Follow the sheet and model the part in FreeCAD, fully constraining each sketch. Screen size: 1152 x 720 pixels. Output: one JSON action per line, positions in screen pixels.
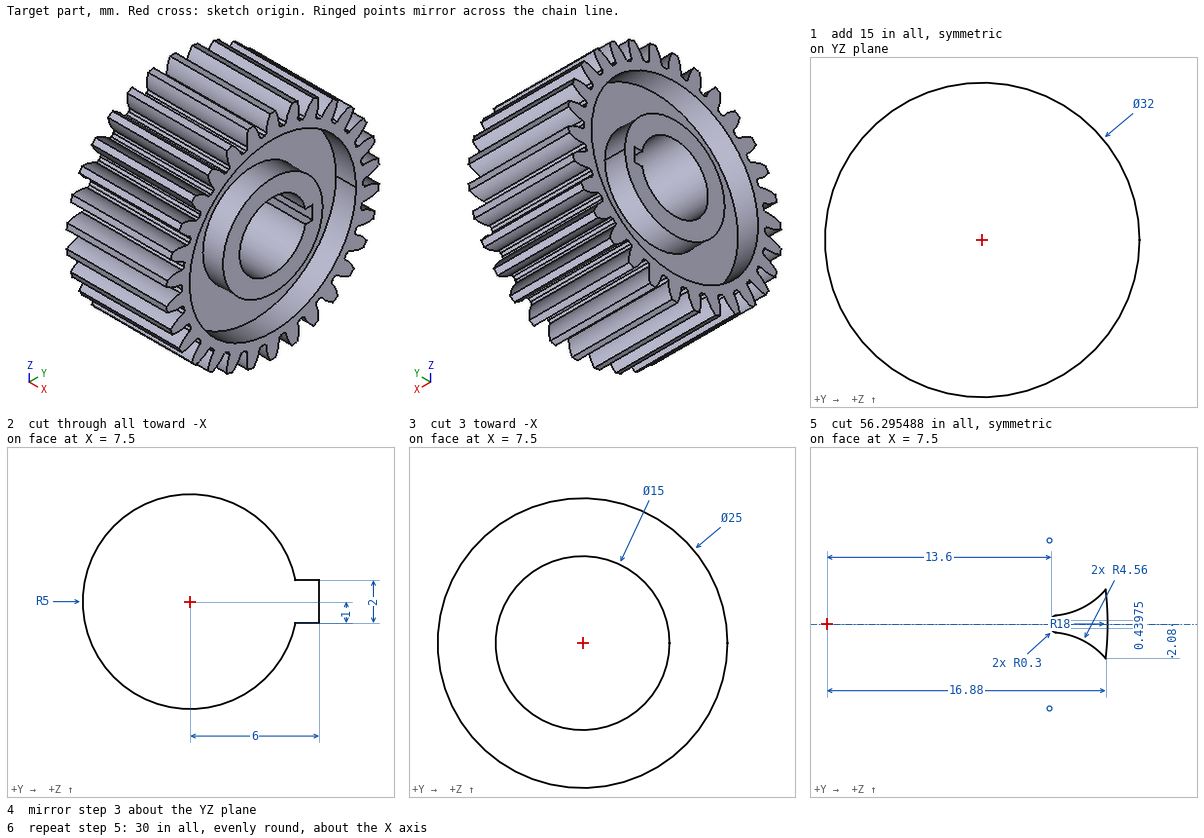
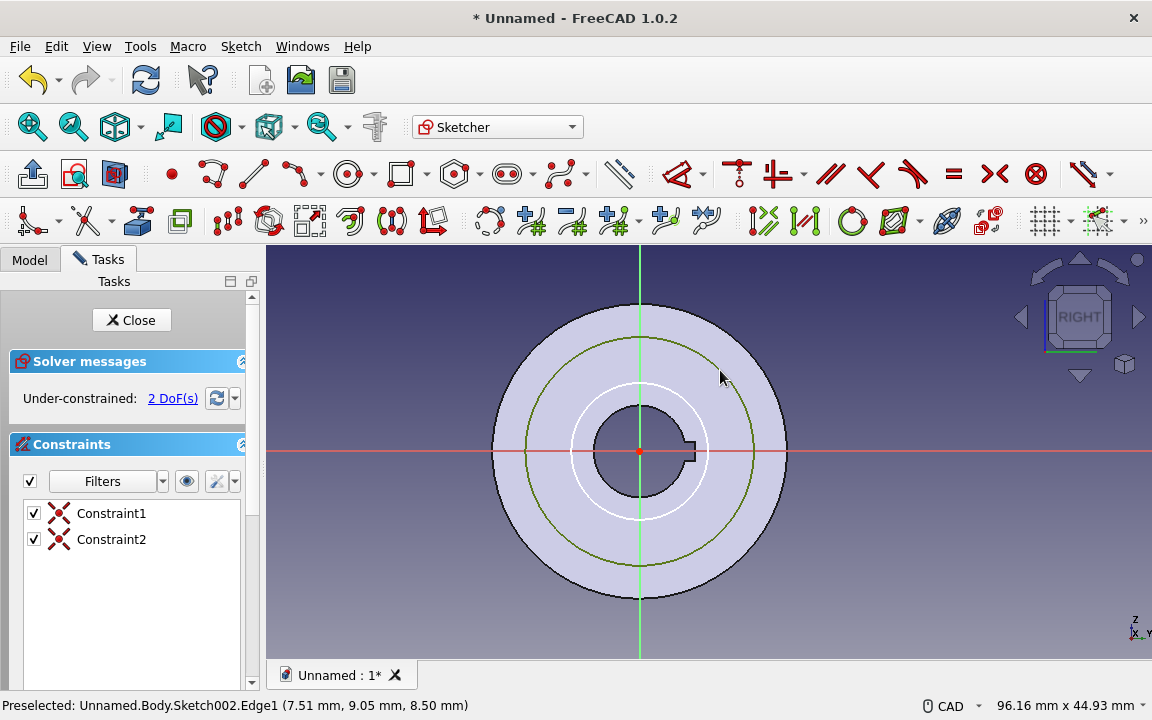
{"action": "left_click", "coordinate": [702, 174]}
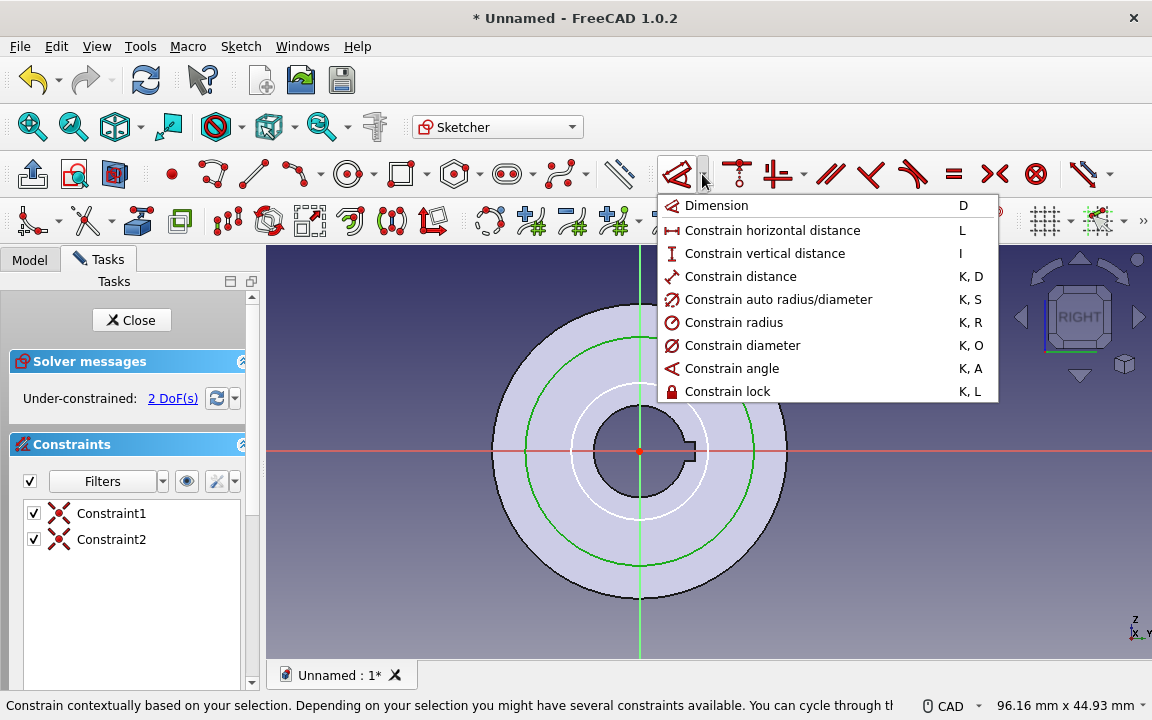
{"action": "left_click", "coordinate": [828, 346]}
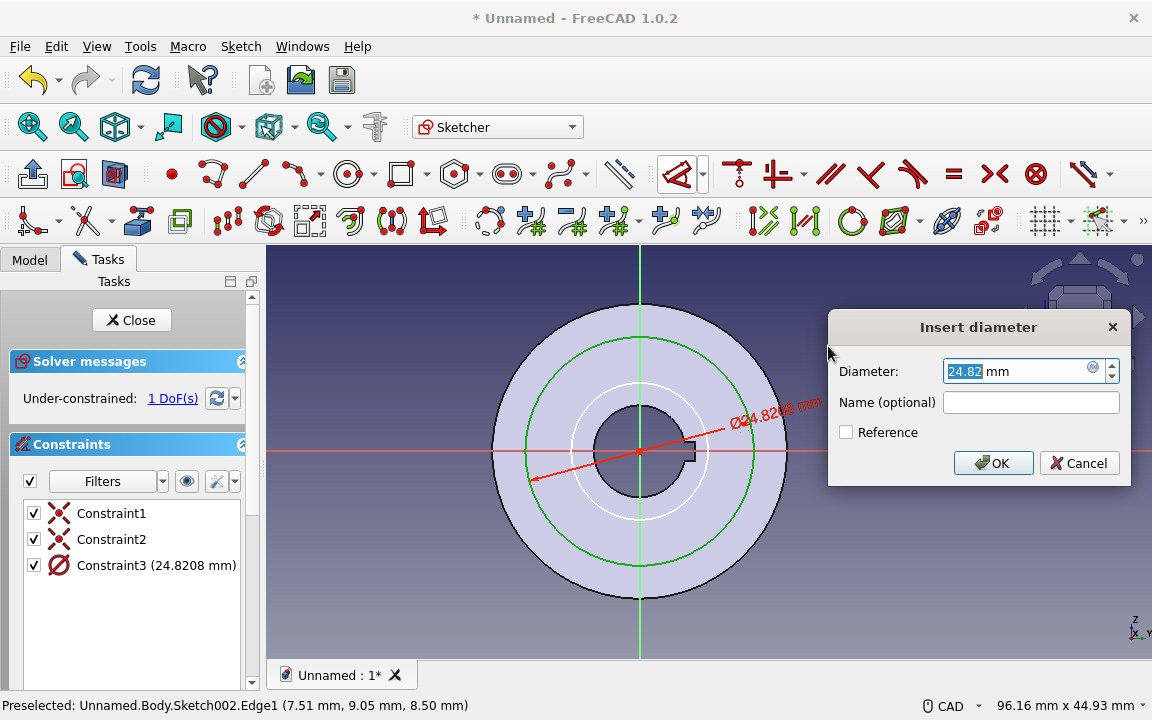
{"action": "type", "text": "25"}
{"action": "key", "text": "Return"}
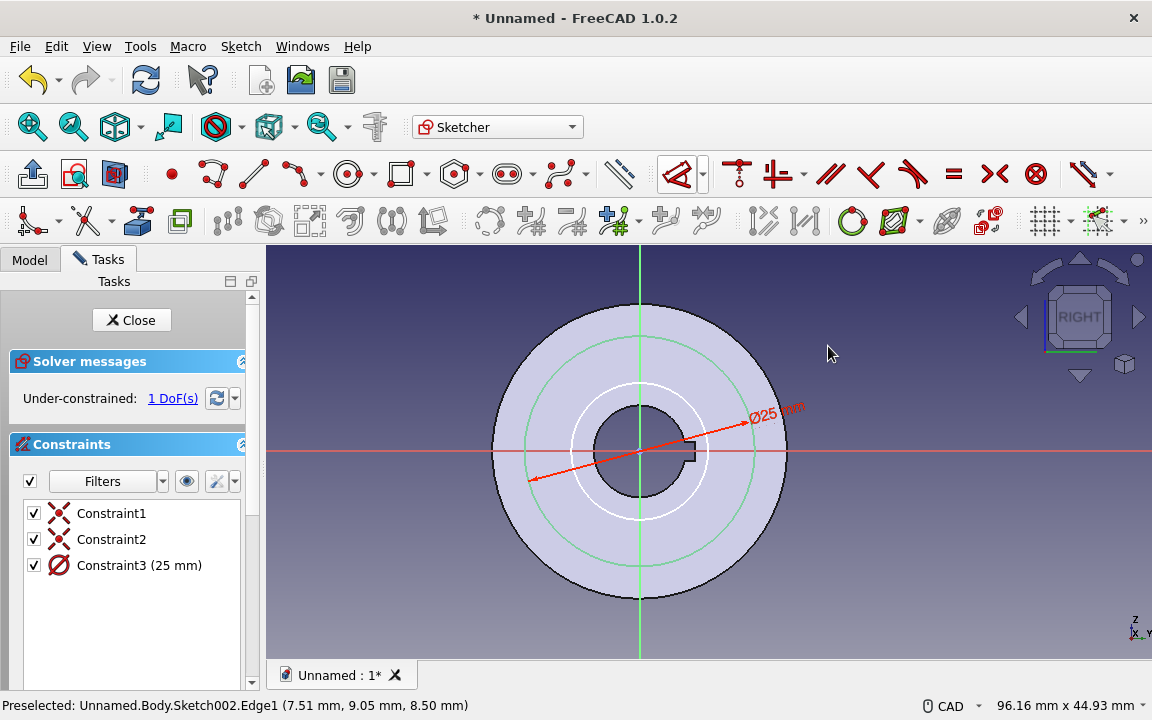
{"action": "left_click", "coordinate": [688, 403]}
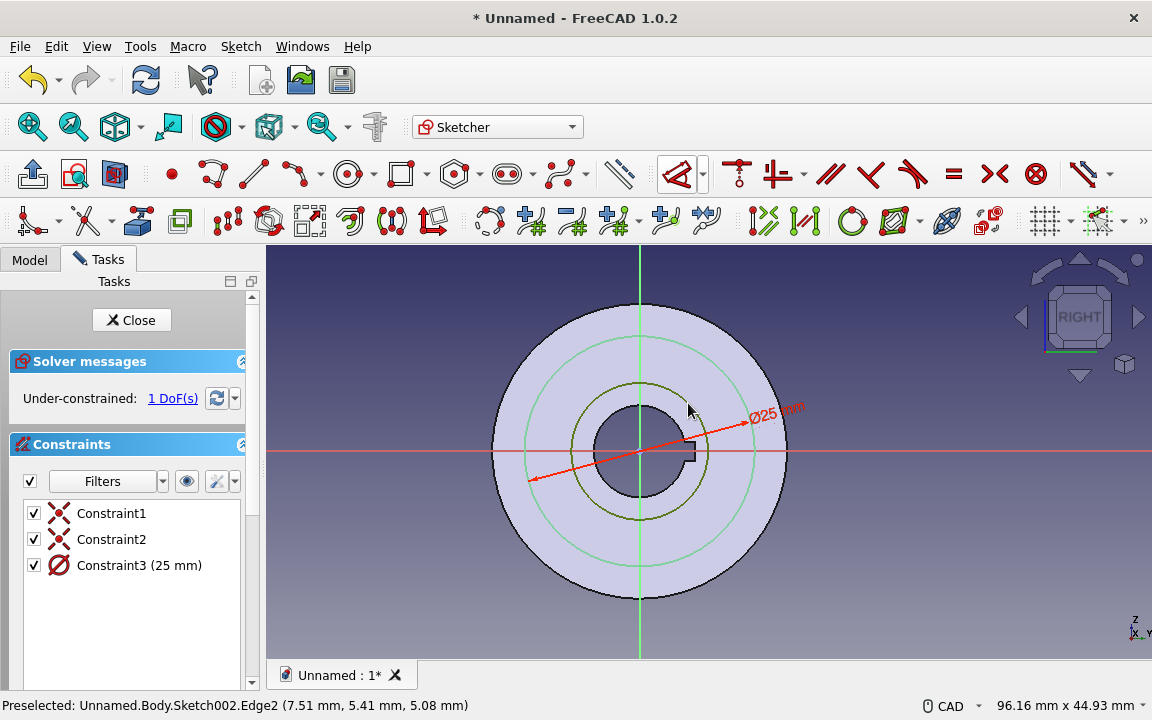
{"action": "left_click", "coordinate": [702, 174]}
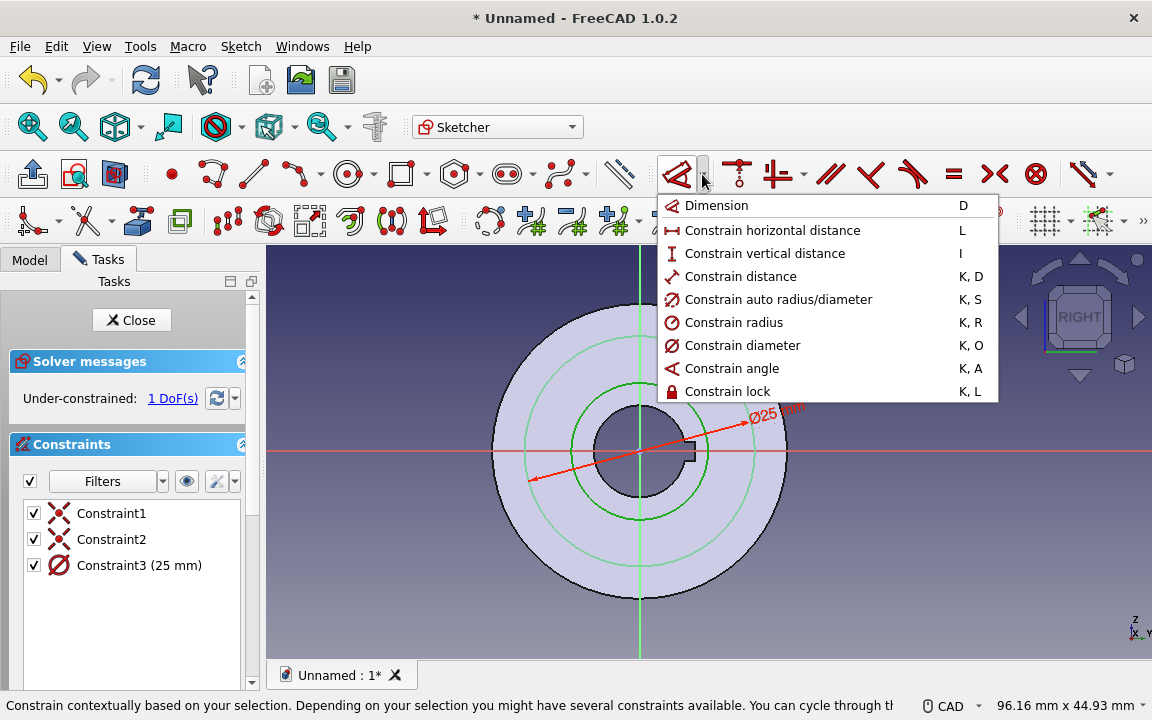
{"action": "left_click", "coordinate": [828, 346]}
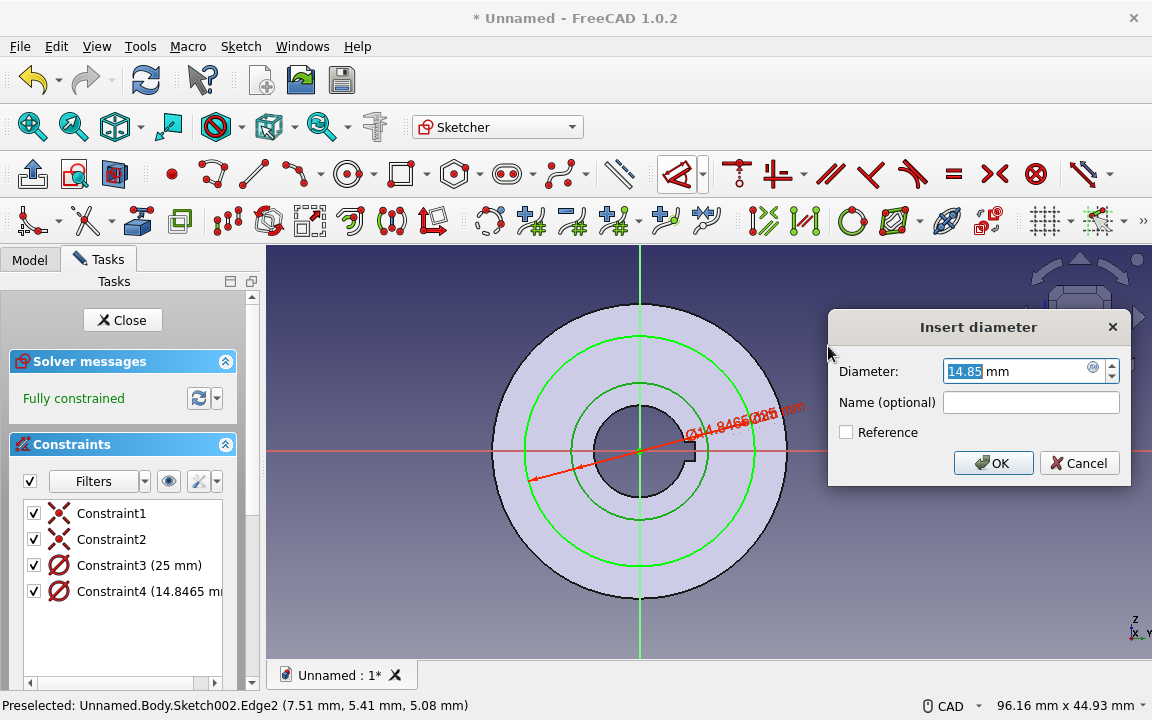
{"action": "type", "text": "15"}
{"action": "key", "text": "Return"}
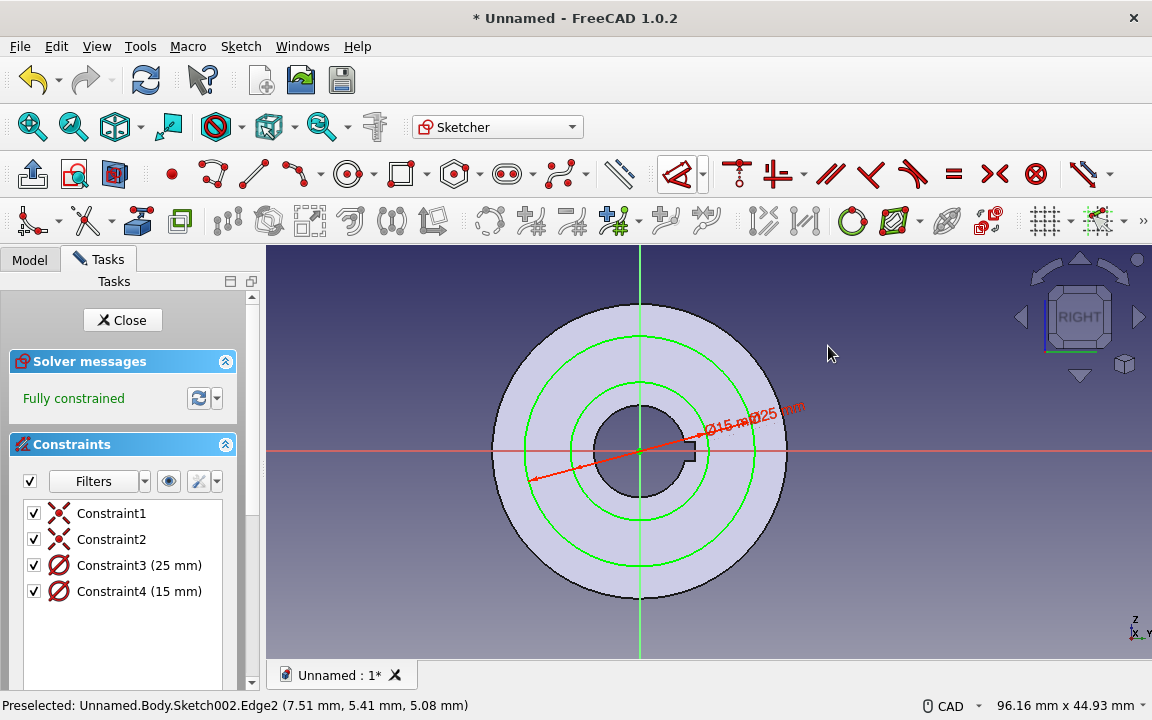
{"action": "left_click", "coordinate": [123, 320]}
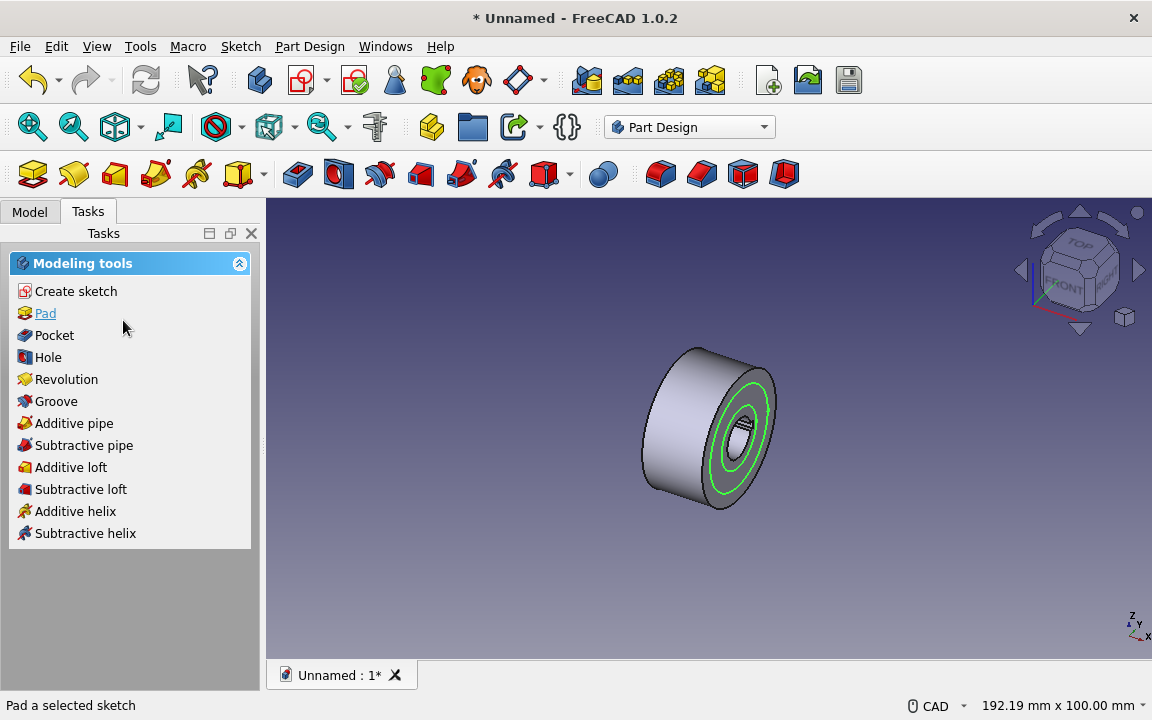
{"action": "left_click", "coordinate": [298, 174]}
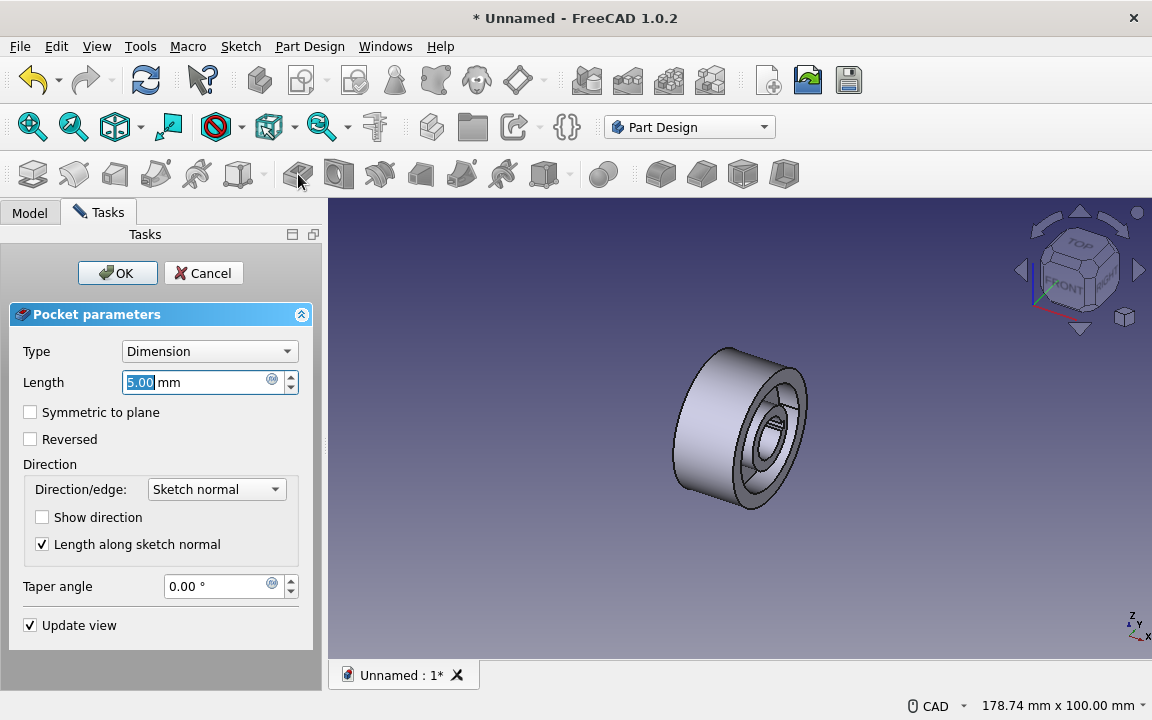
{"action": "type", "text": "3"}
{"action": "key", "text": "Tab"}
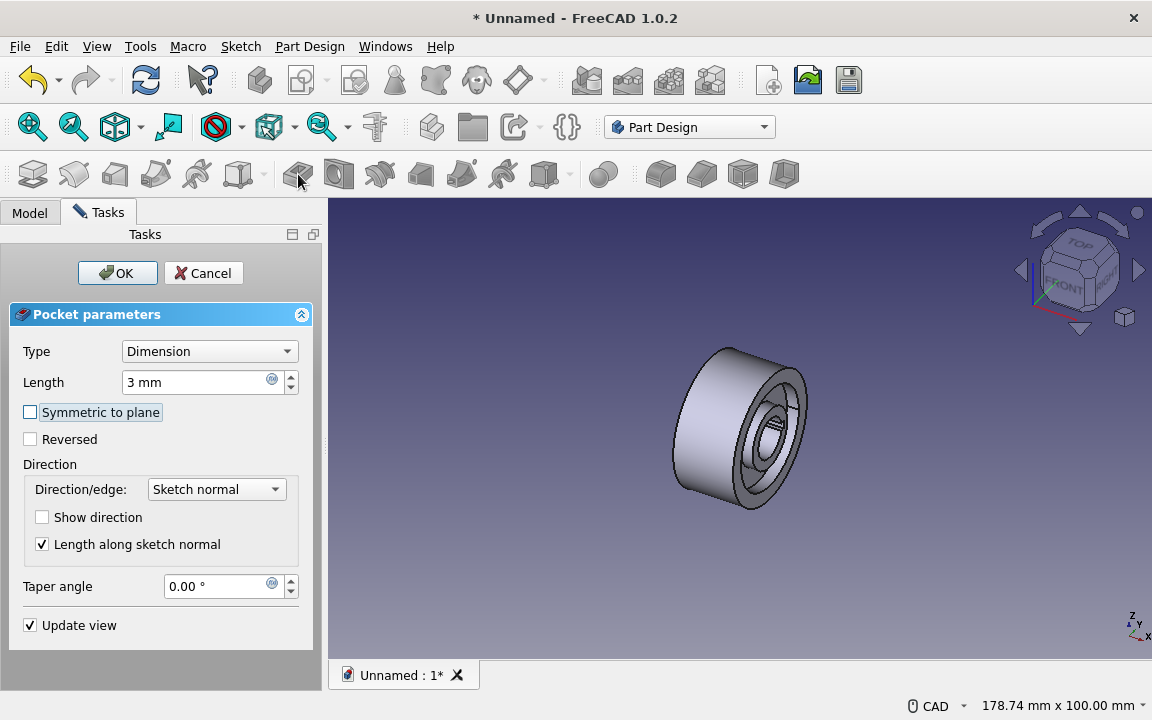
{"action": "left_click", "coordinate": [118, 273]}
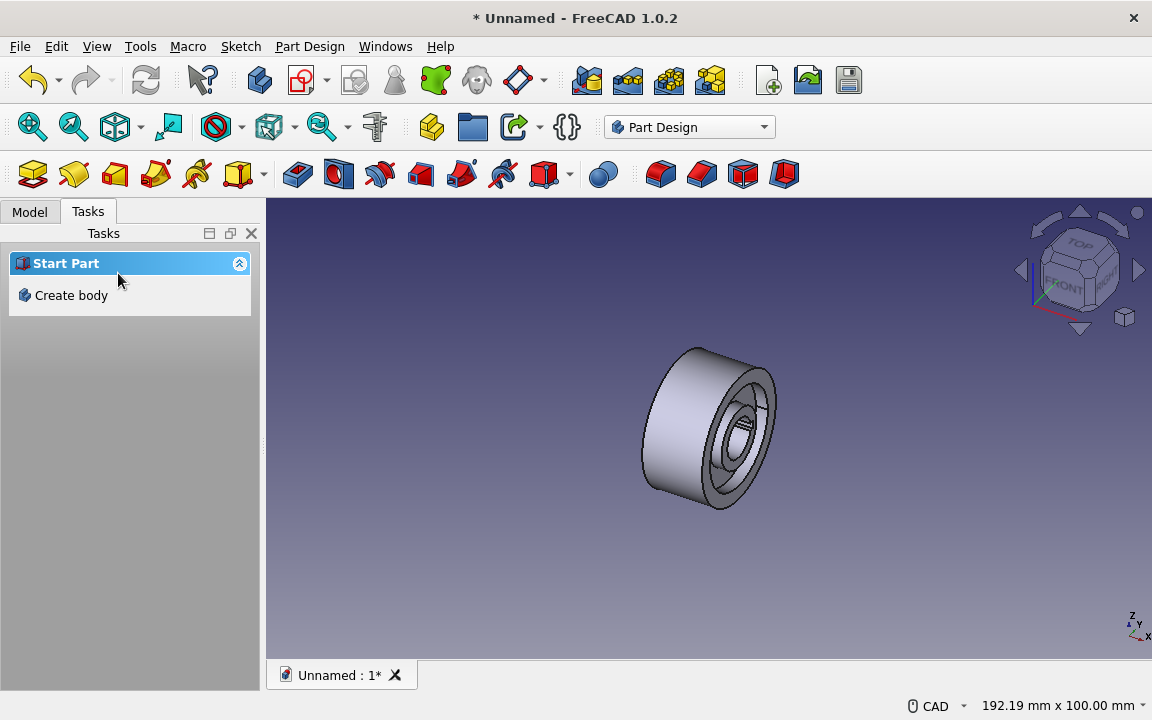
{"action": "left_click", "coordinate": [30, 212]}